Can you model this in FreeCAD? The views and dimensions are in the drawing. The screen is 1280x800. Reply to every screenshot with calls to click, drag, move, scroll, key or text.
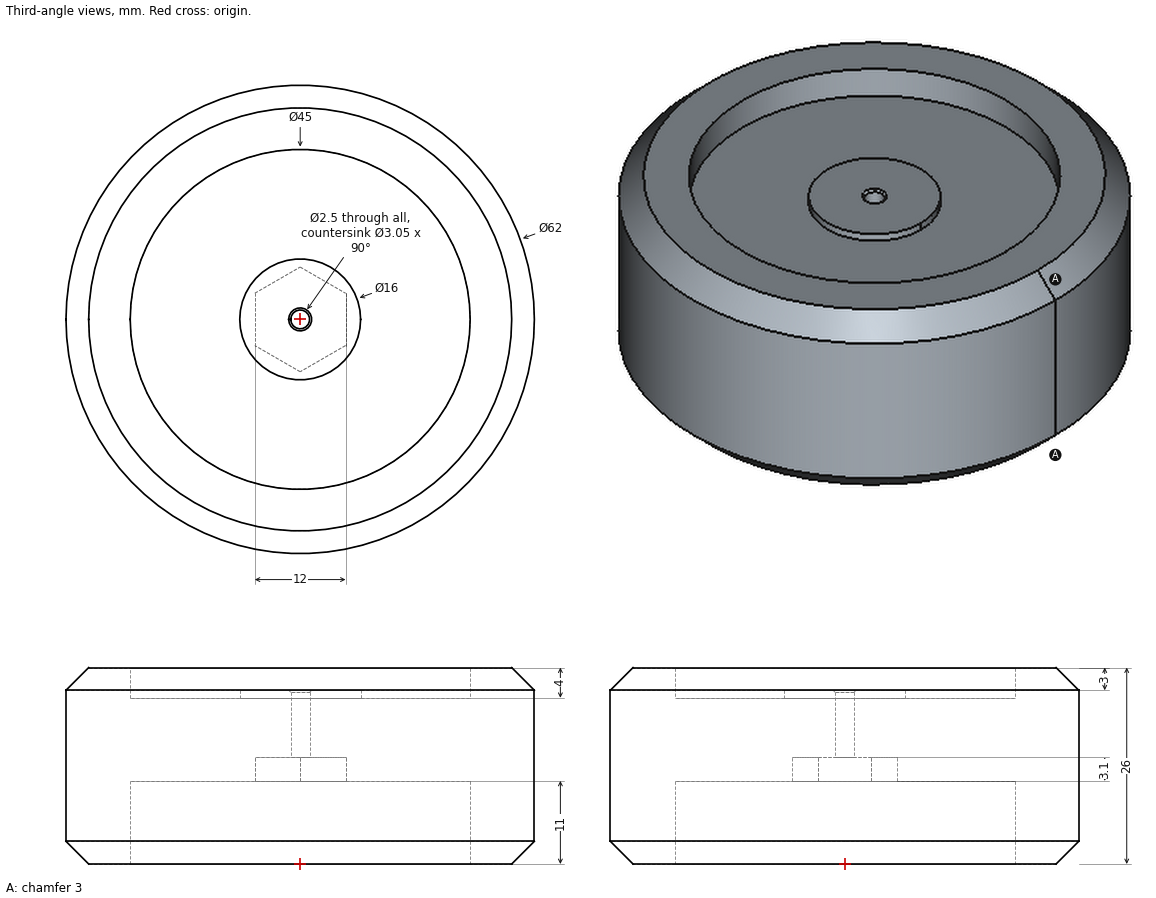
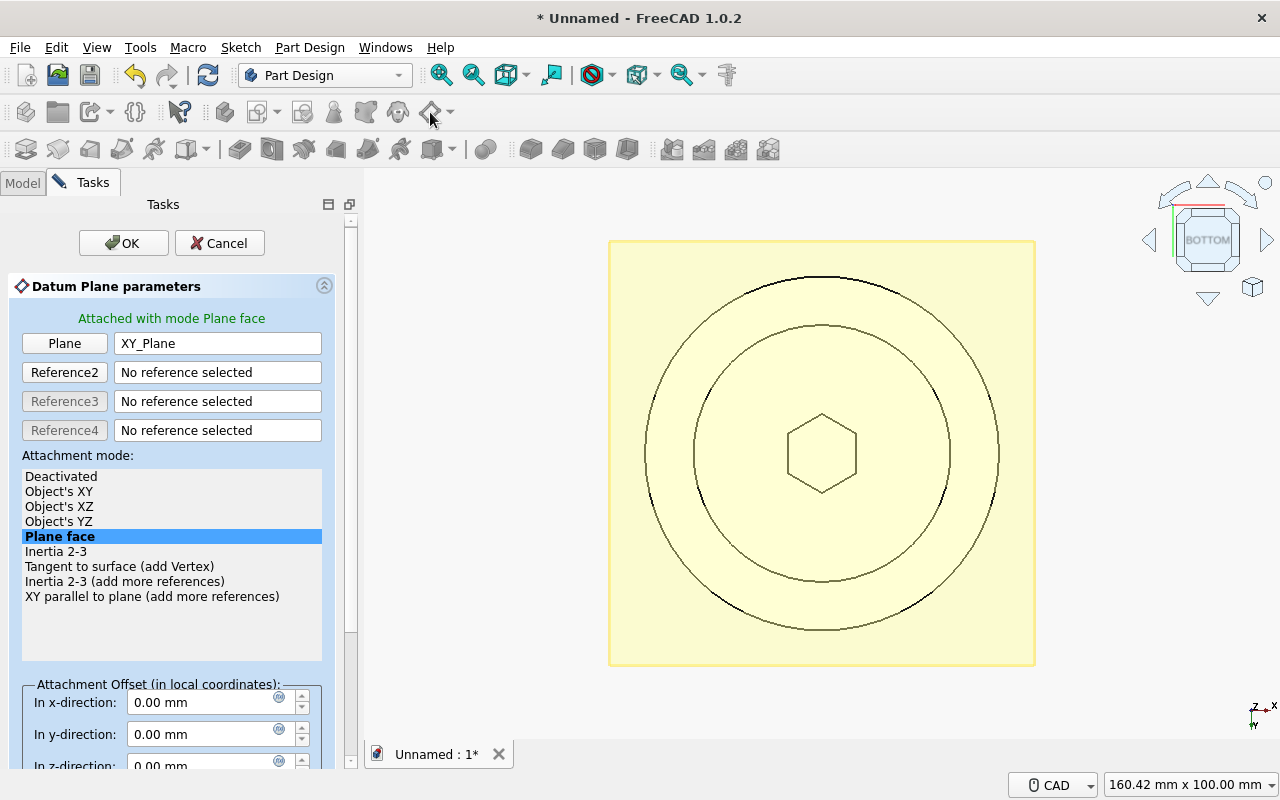
scroll(351, 491, down, 2)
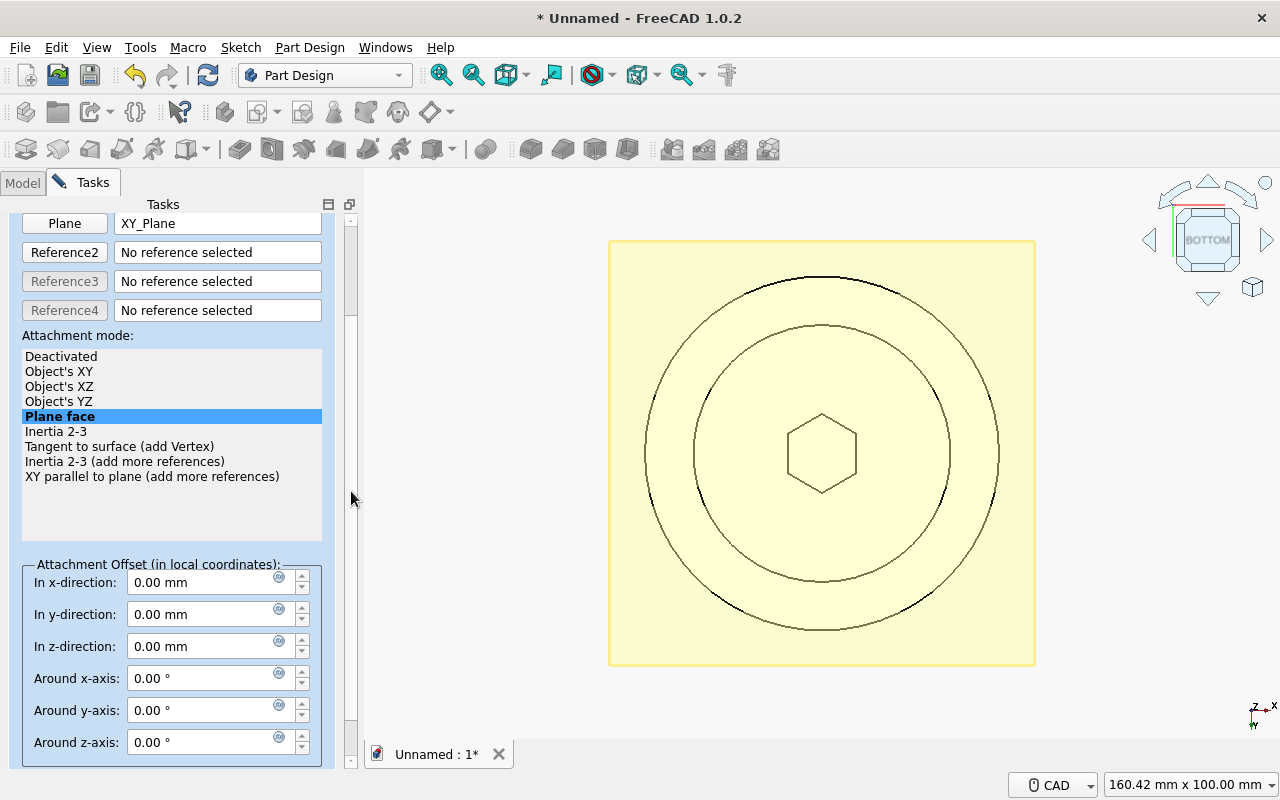
triple_click(210, 646)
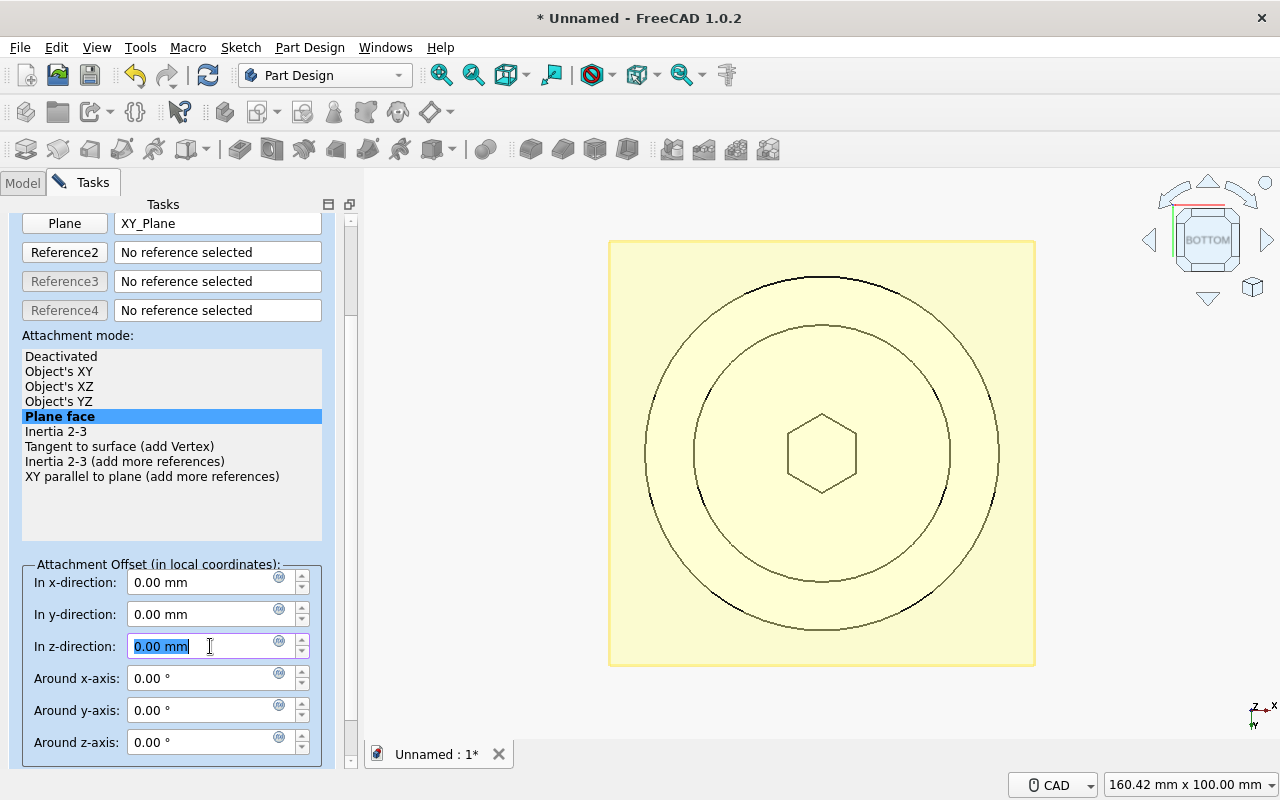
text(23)
key(Tab)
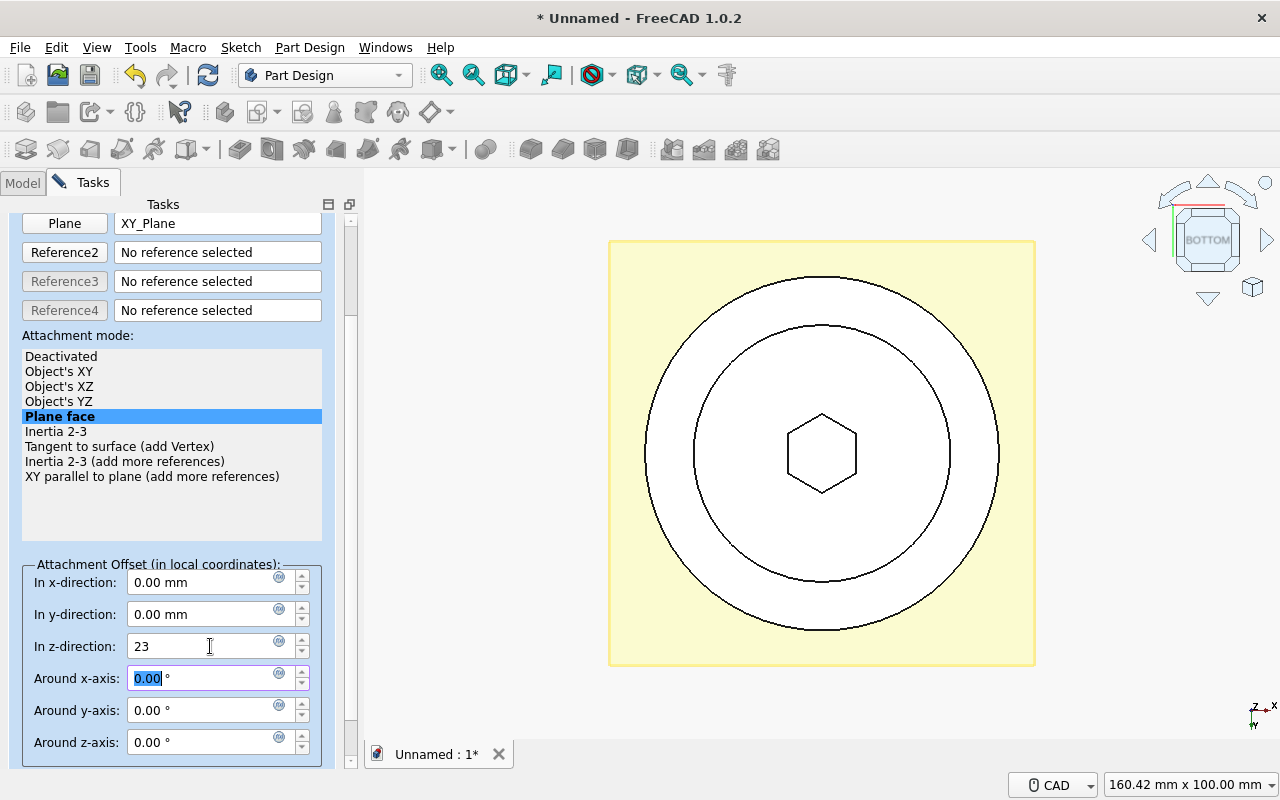
scroll(351, 491, up, 3)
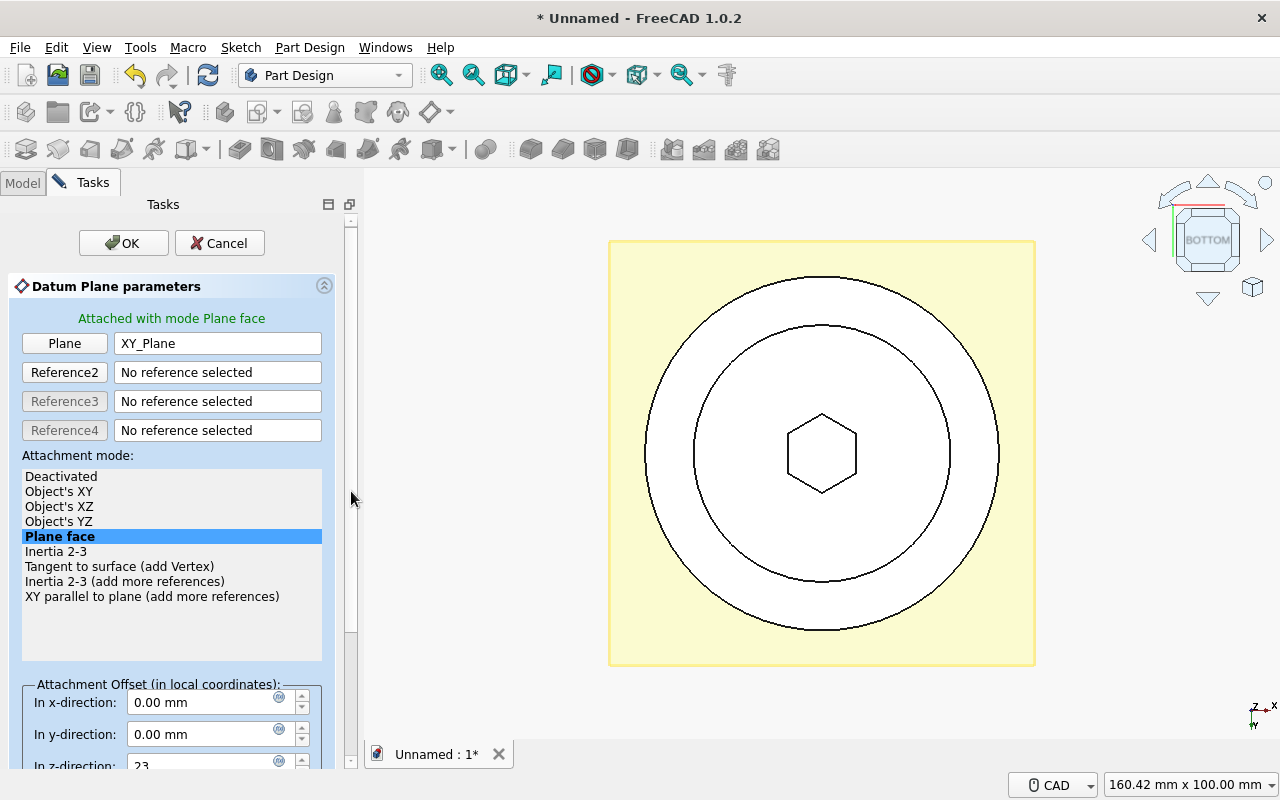
click(124, 243)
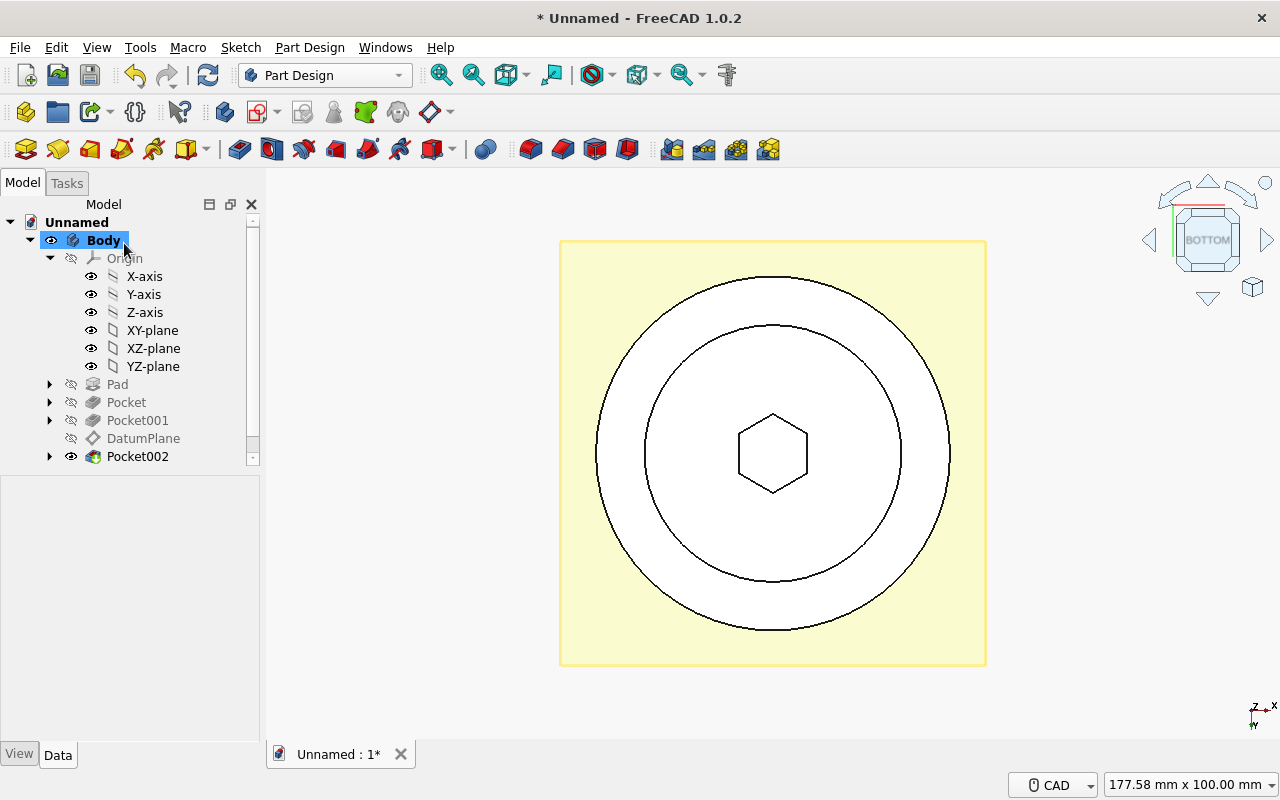
scroll(100, 344, down, 3)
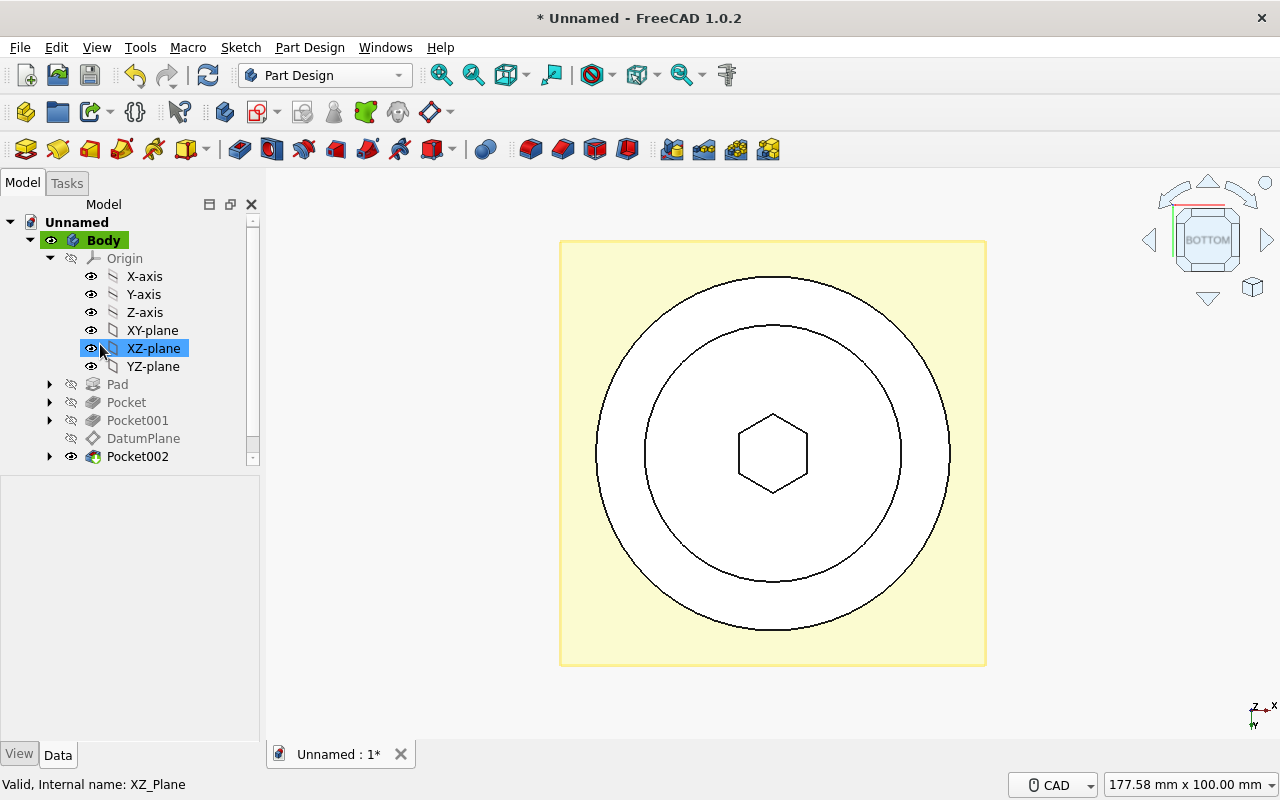
click(116, 456)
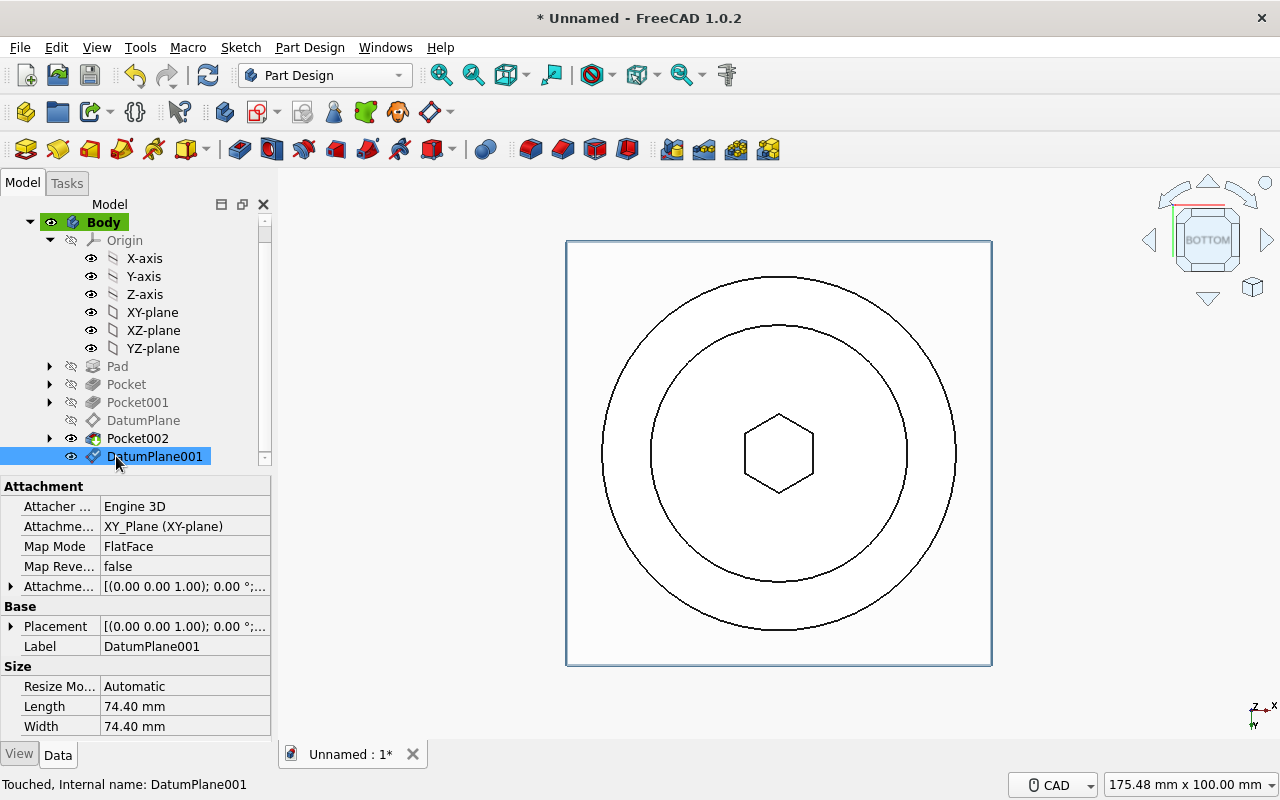
click(258, 112)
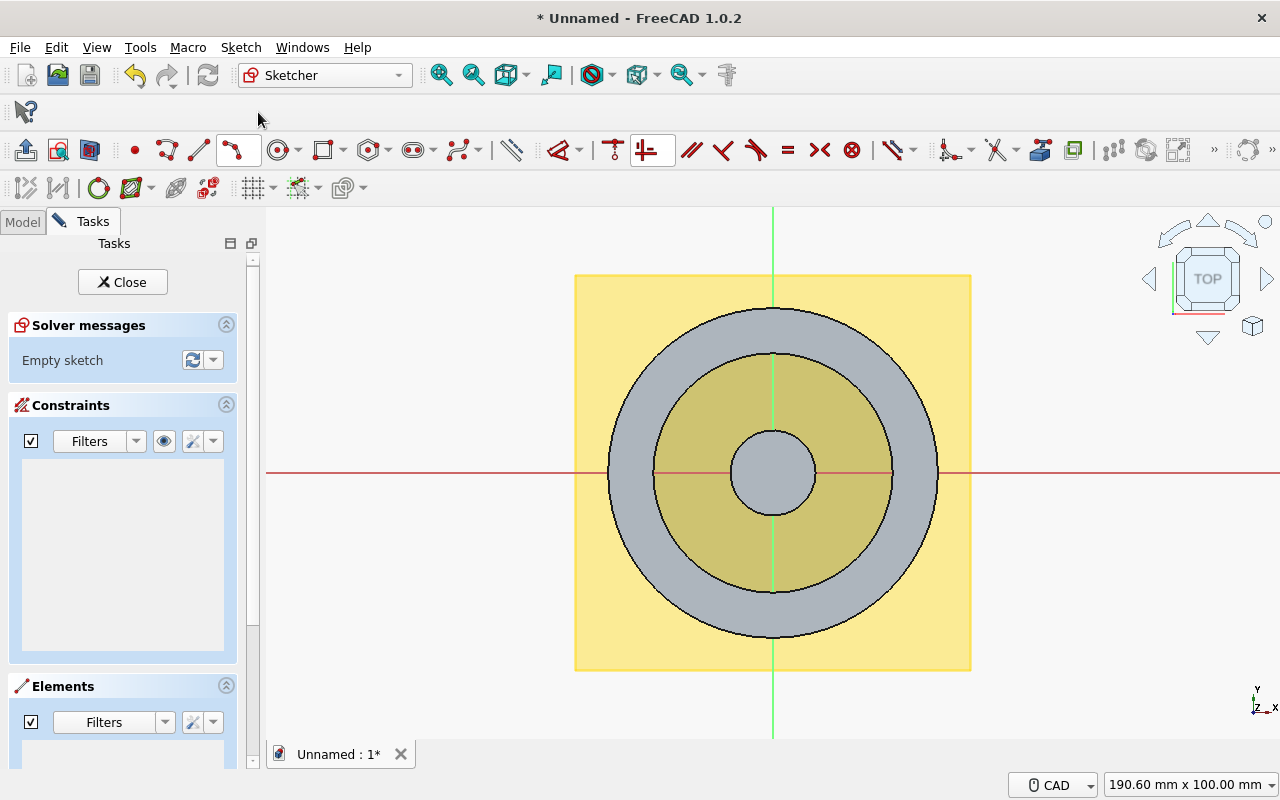
click(90, 150)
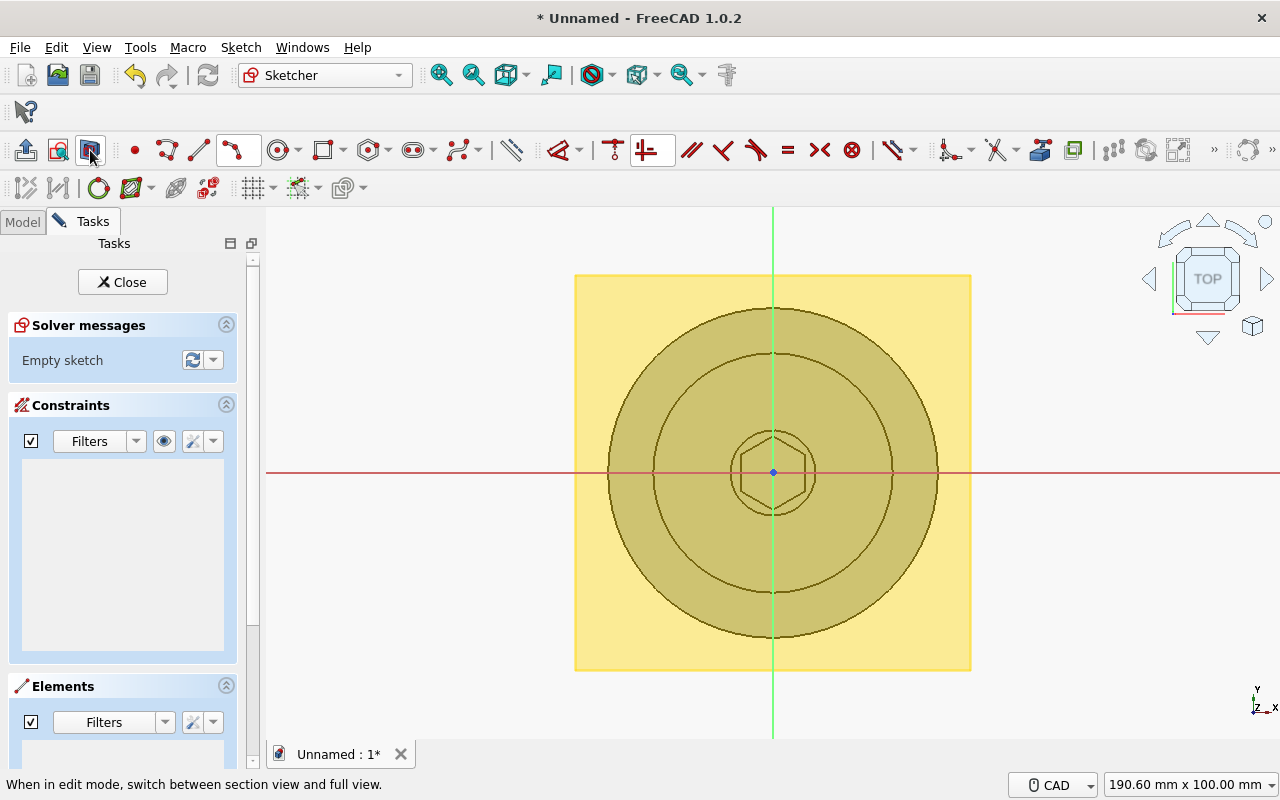
scroll(795, 473, up, 7)